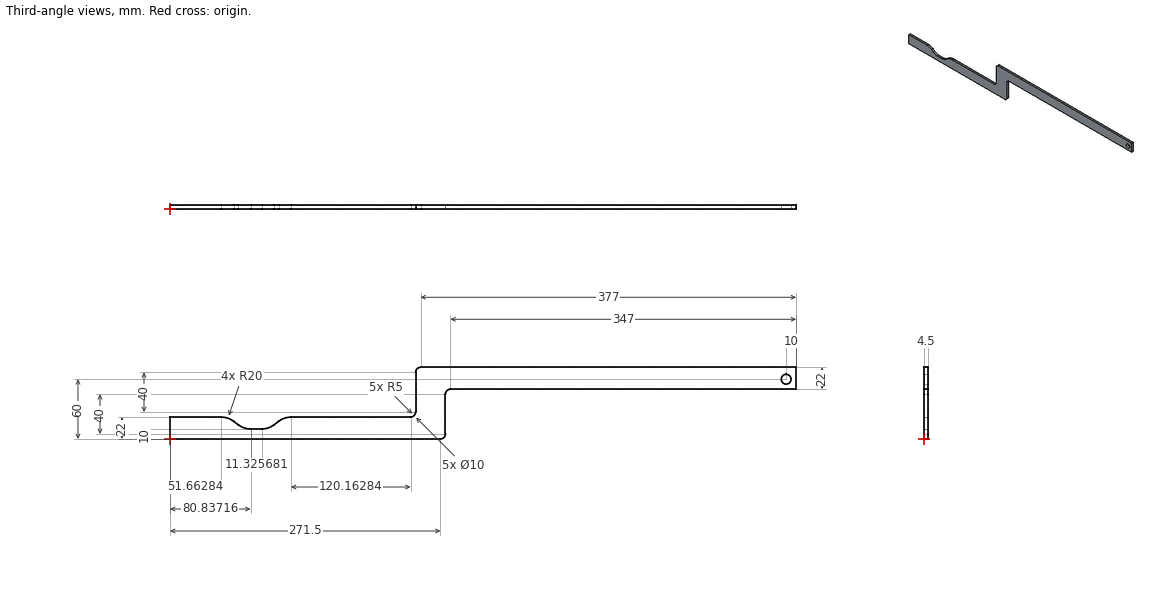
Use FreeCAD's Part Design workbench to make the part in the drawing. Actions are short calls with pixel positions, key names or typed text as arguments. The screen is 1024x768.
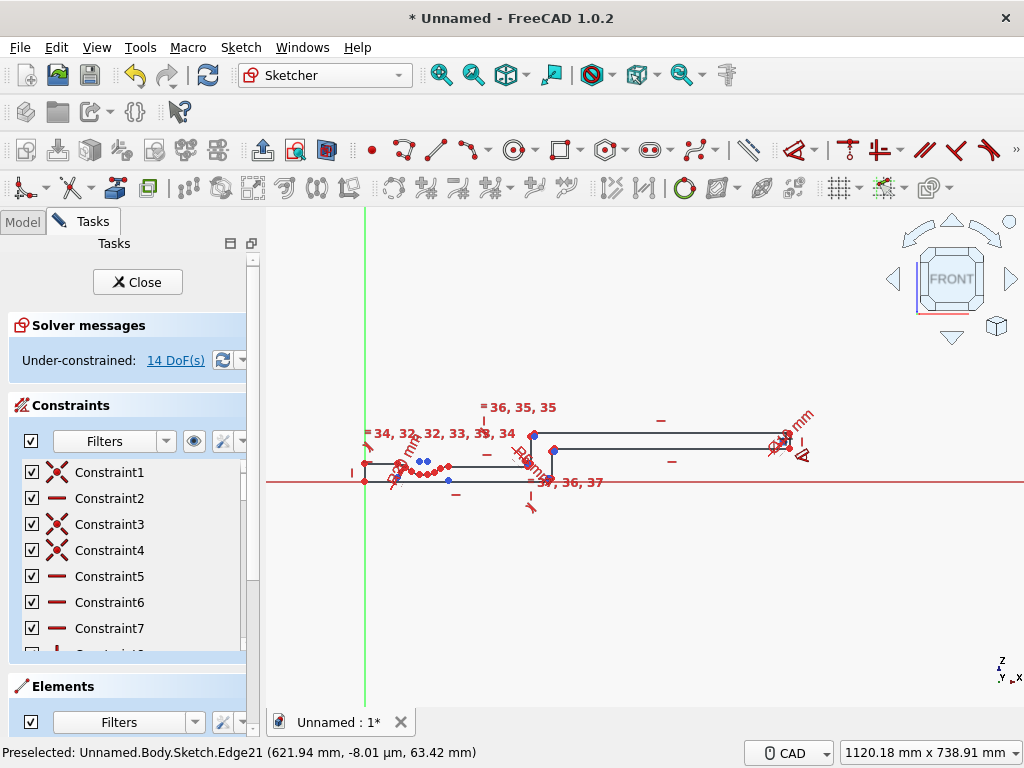
scroll(365, 477, up, 5)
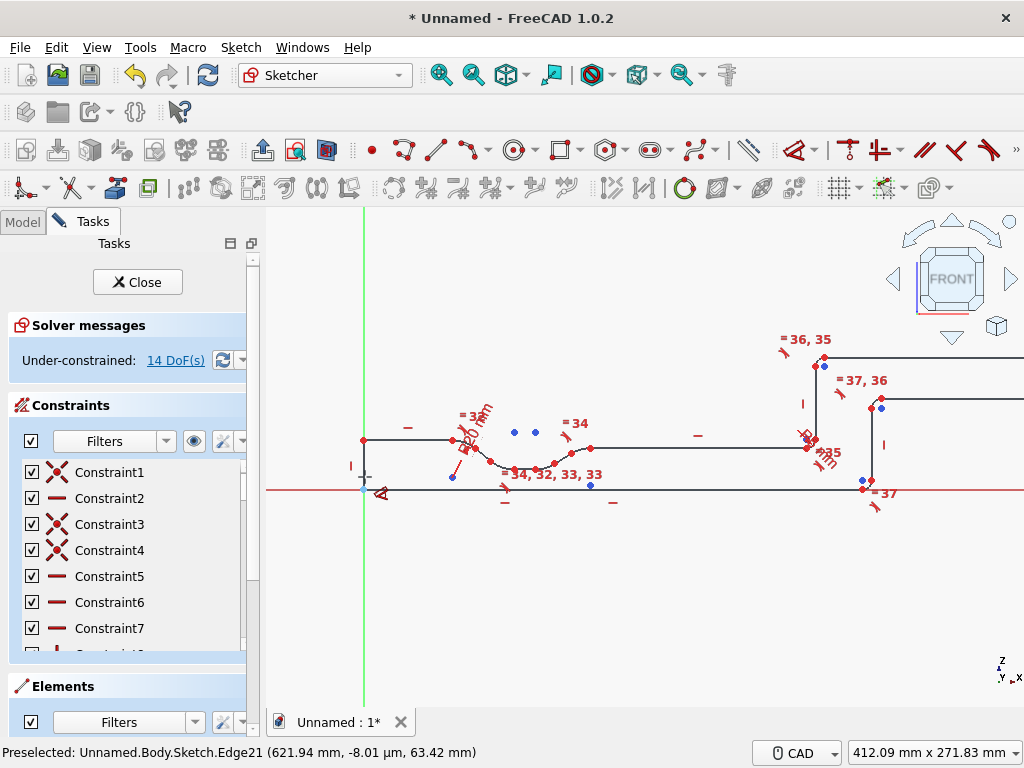
click(364, 475)
click(330, 465)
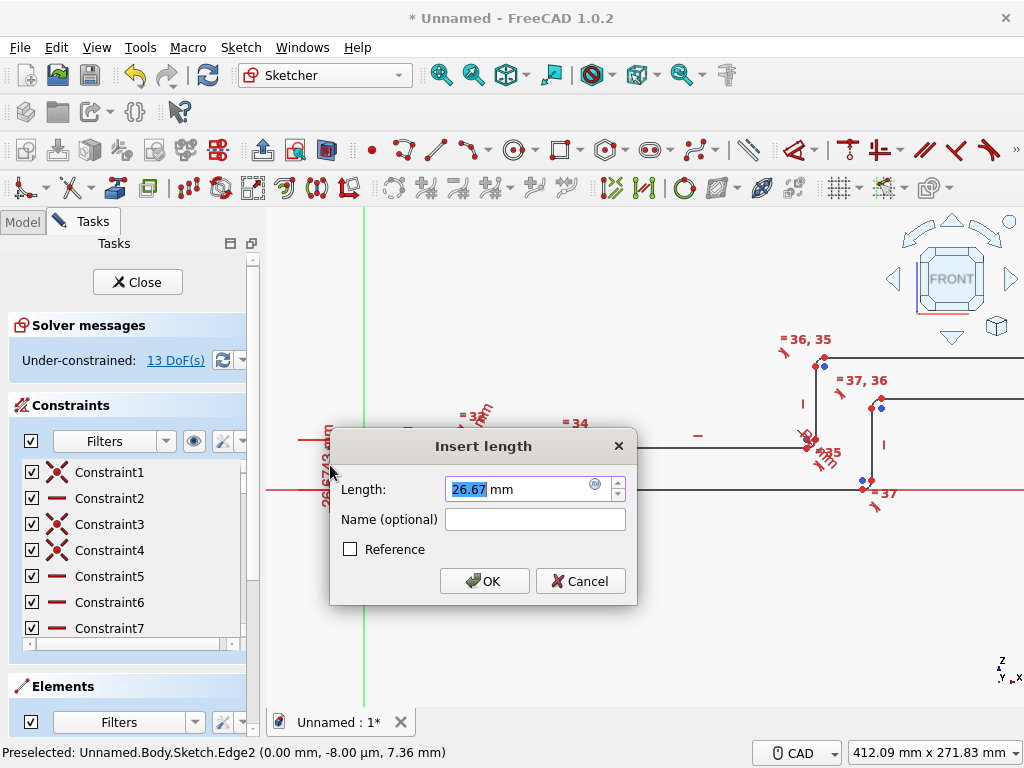
text(22)
key(Return)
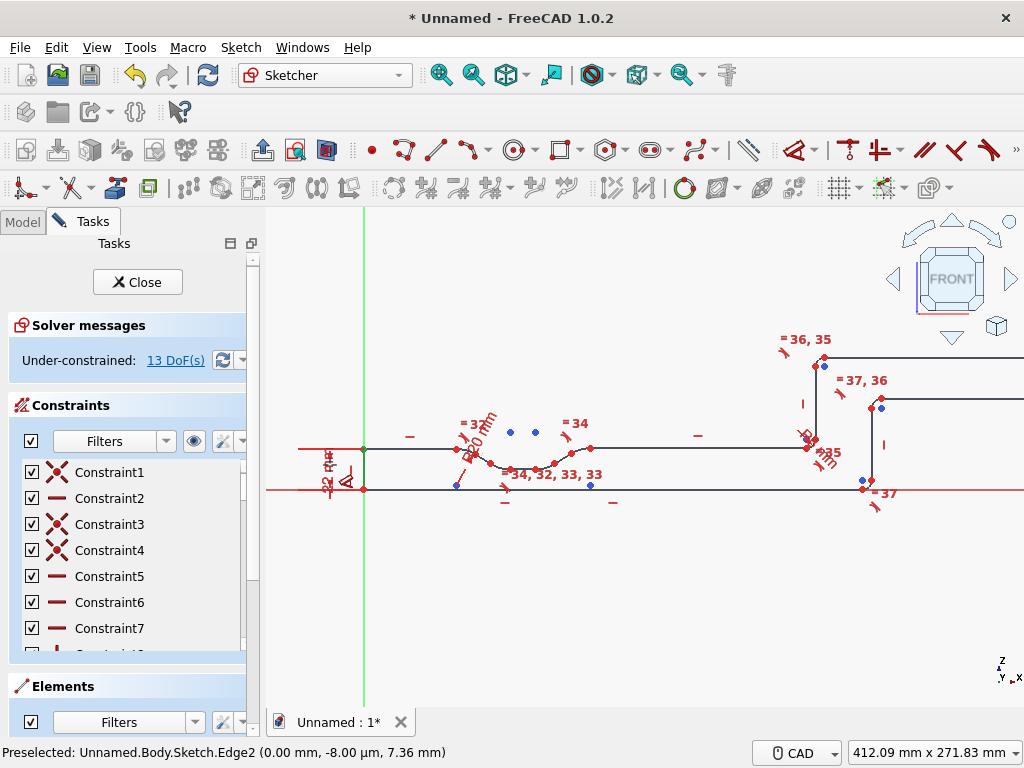
click(816, 417)
click(782, 403)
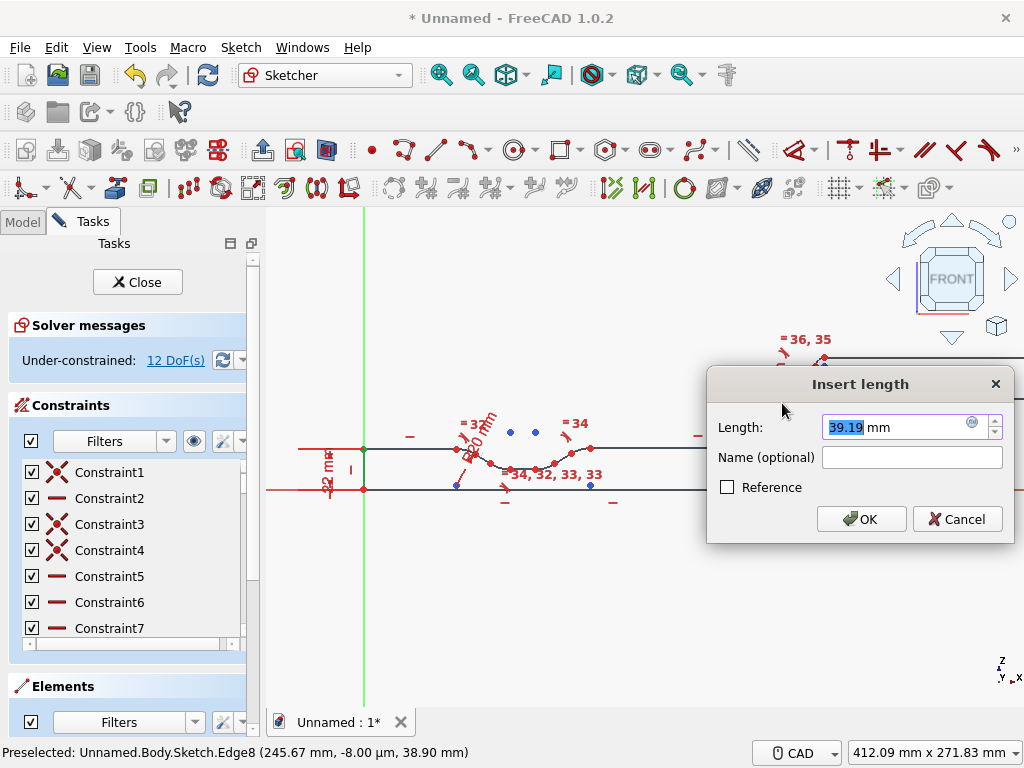
text(40)
key(Return)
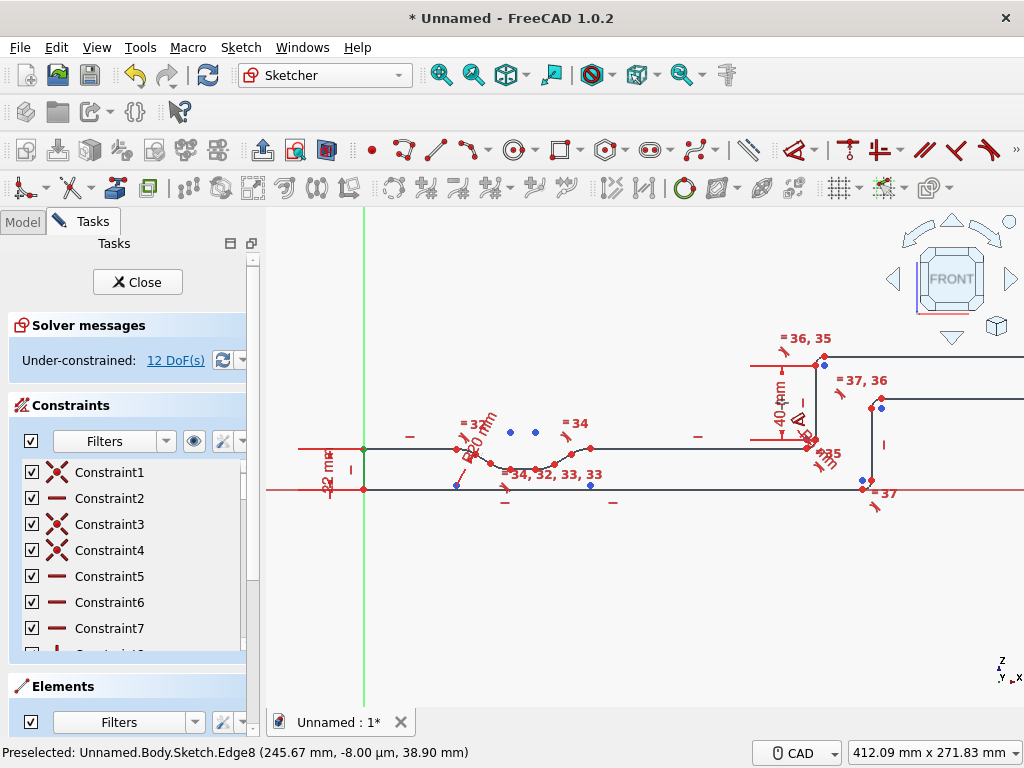
scroll(364, 477, down, 5)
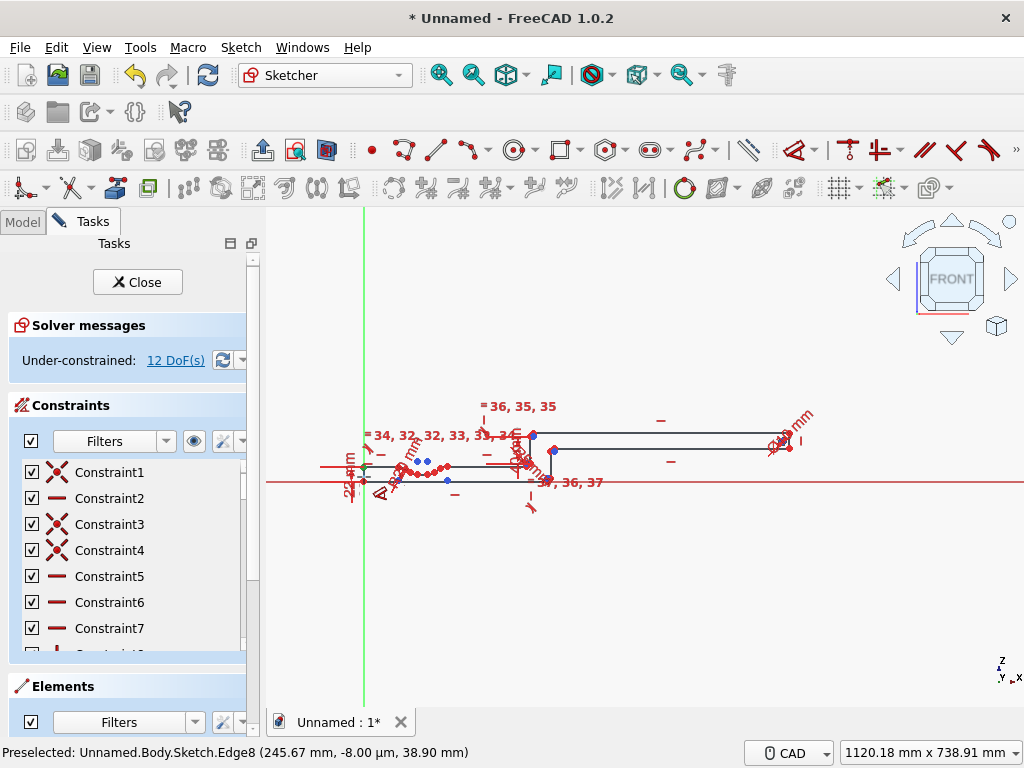
scroll(789, 438, up, 6)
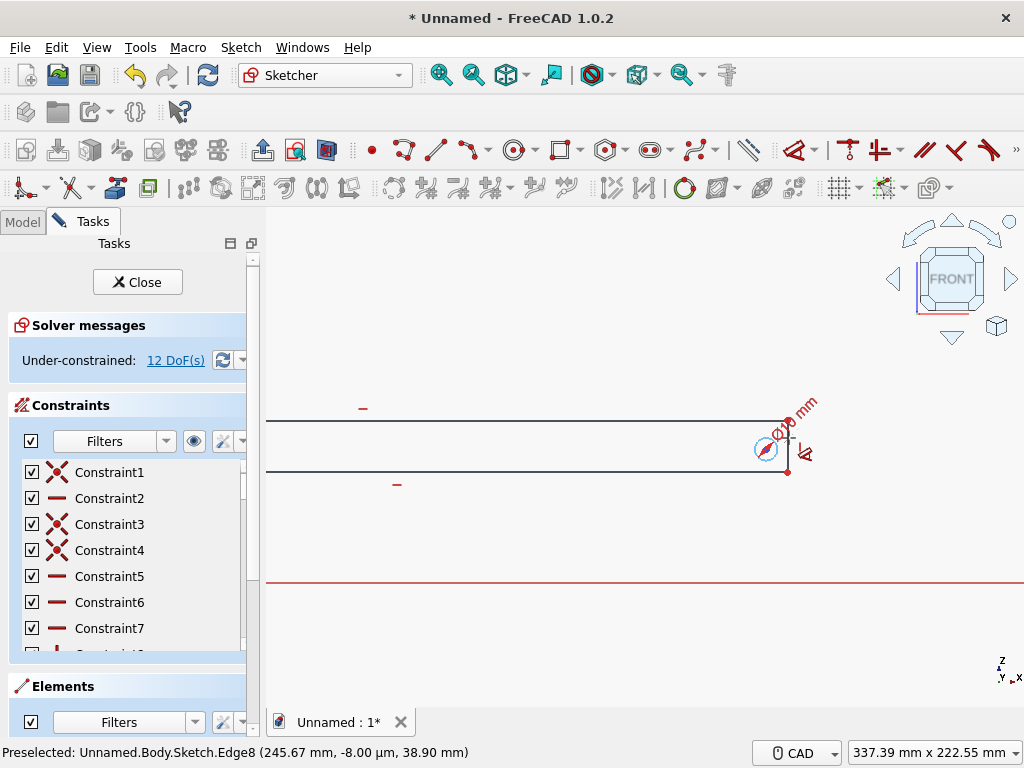
click(788, 436)
click(822, 446)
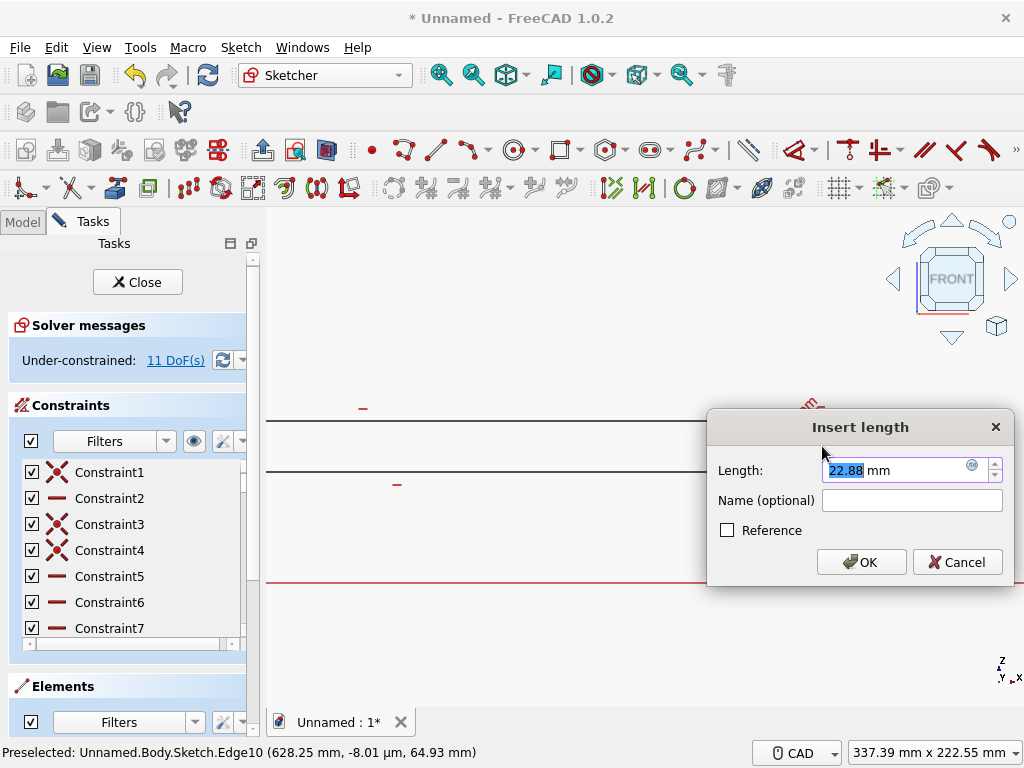
text(22)
key(Return)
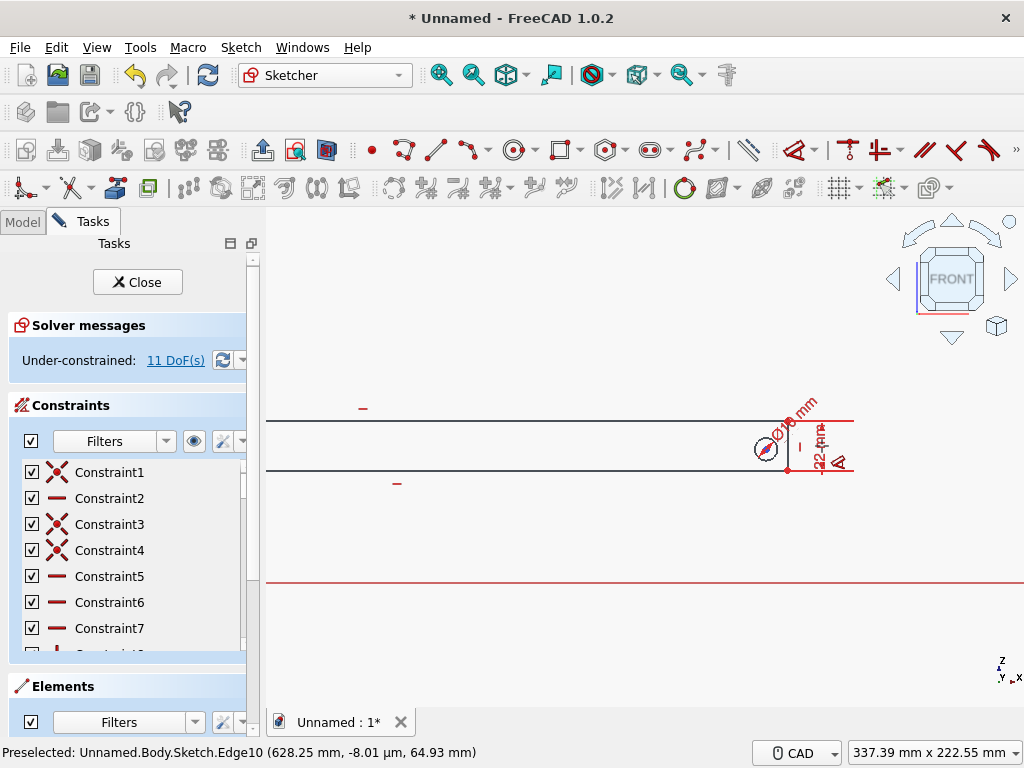
scroll(790, 438, down, 6)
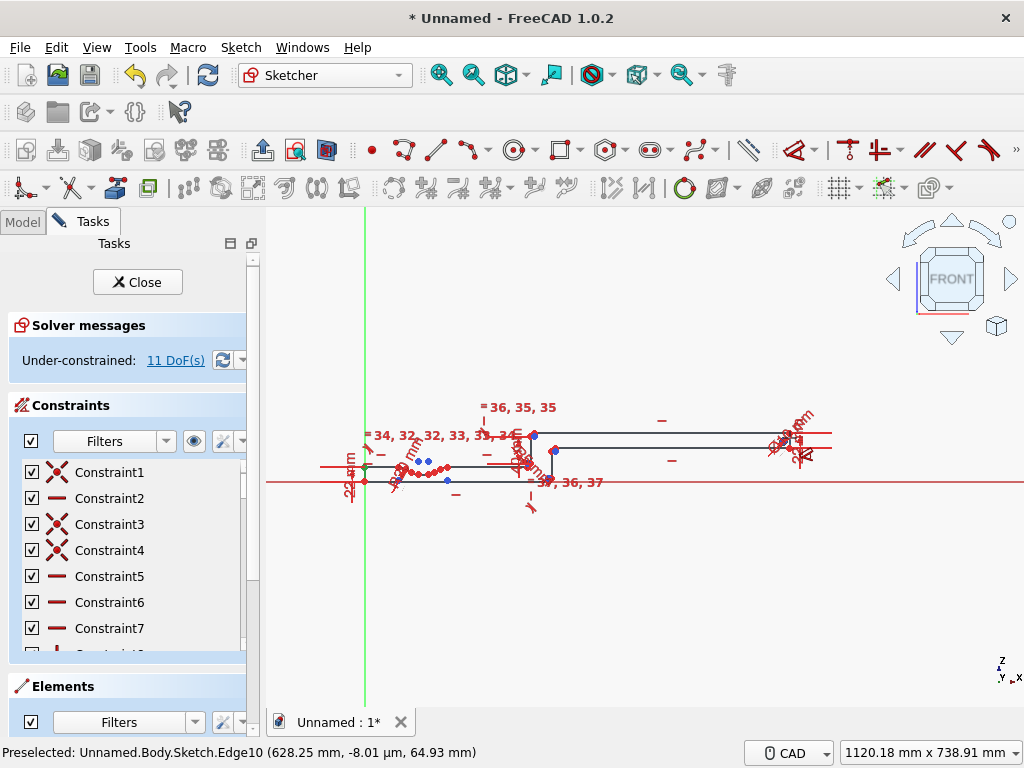
scroll(552, 460, up, 3)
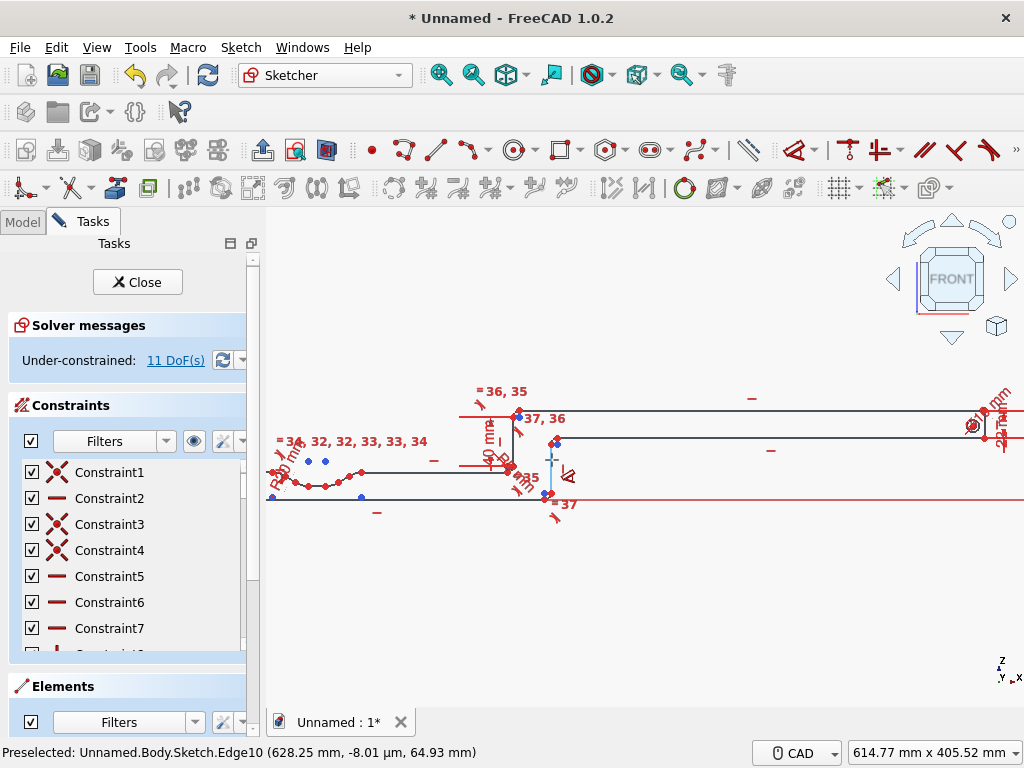
click(551, 459)
click(585, 469)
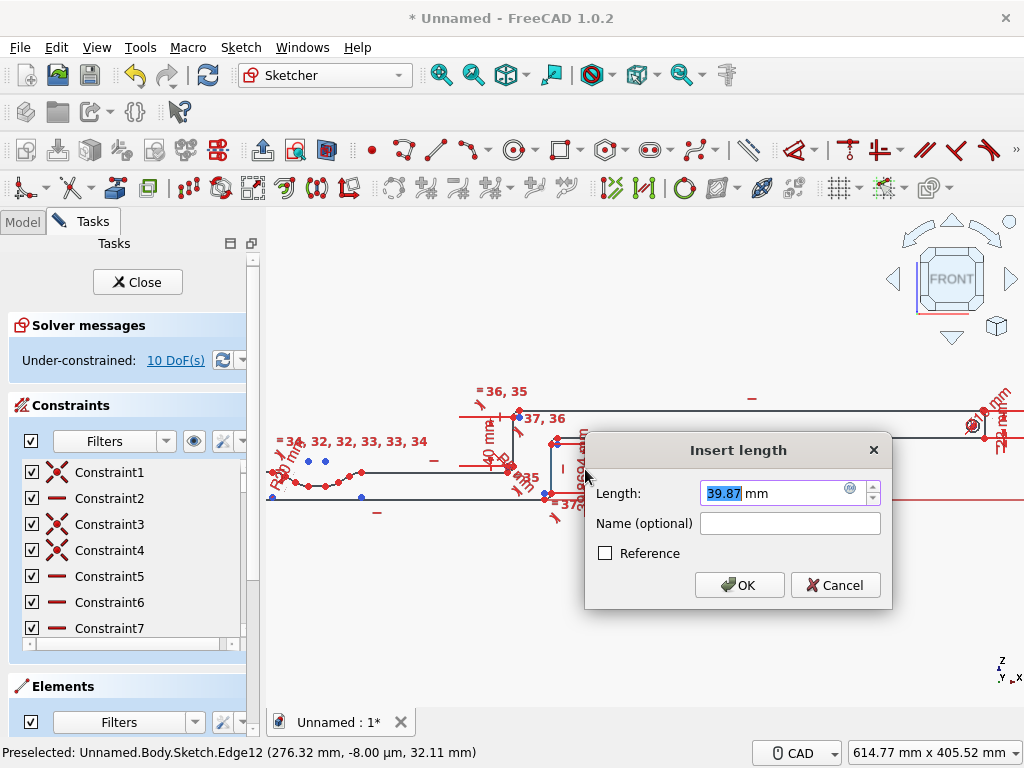
text(40)
key(Return)